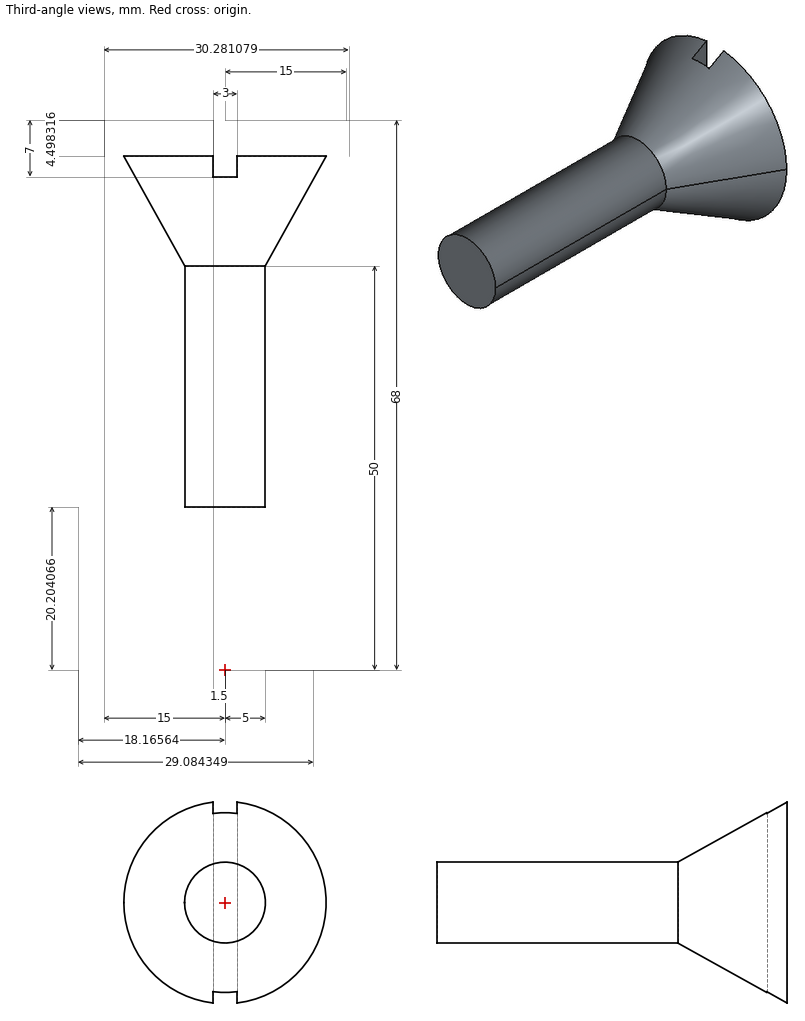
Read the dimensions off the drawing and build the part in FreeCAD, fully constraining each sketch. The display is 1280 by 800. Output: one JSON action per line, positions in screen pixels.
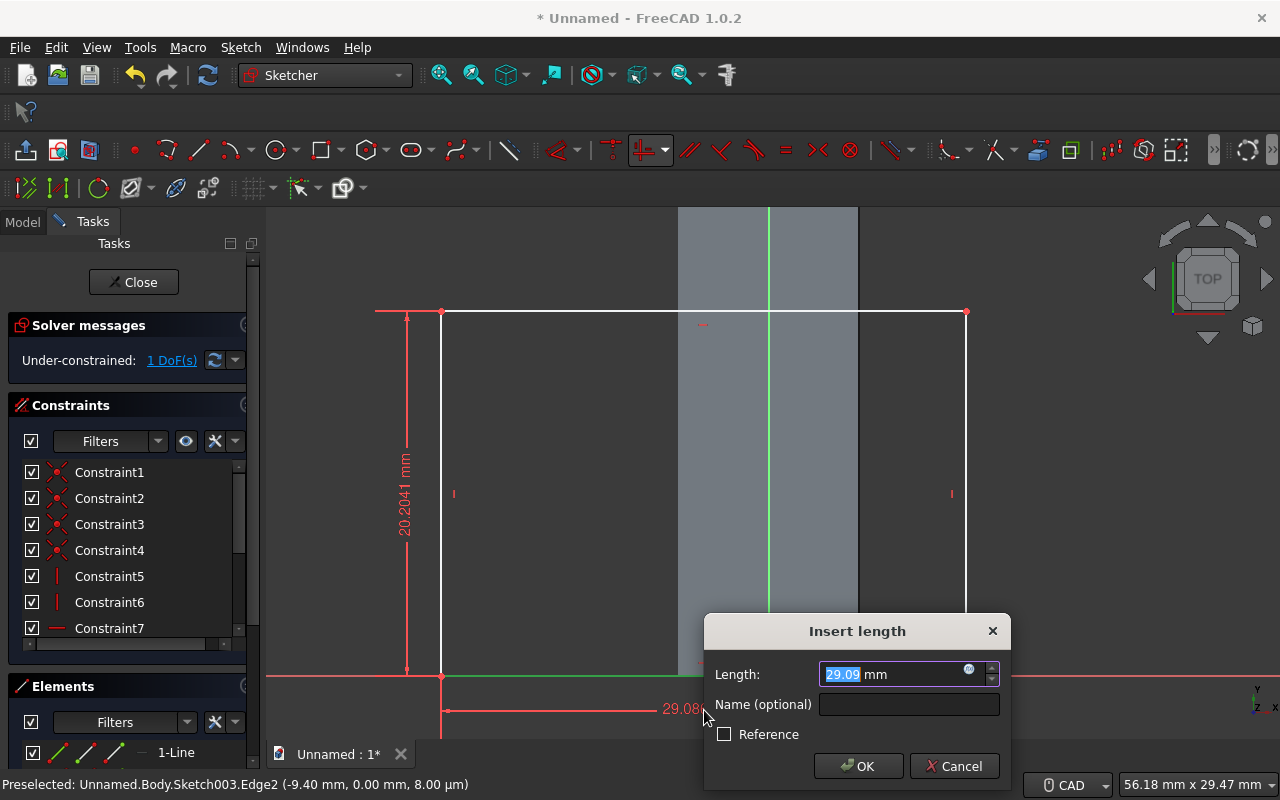
{"action": "type", "text": "29.084349"}
{"action": "key", "text": "Return"}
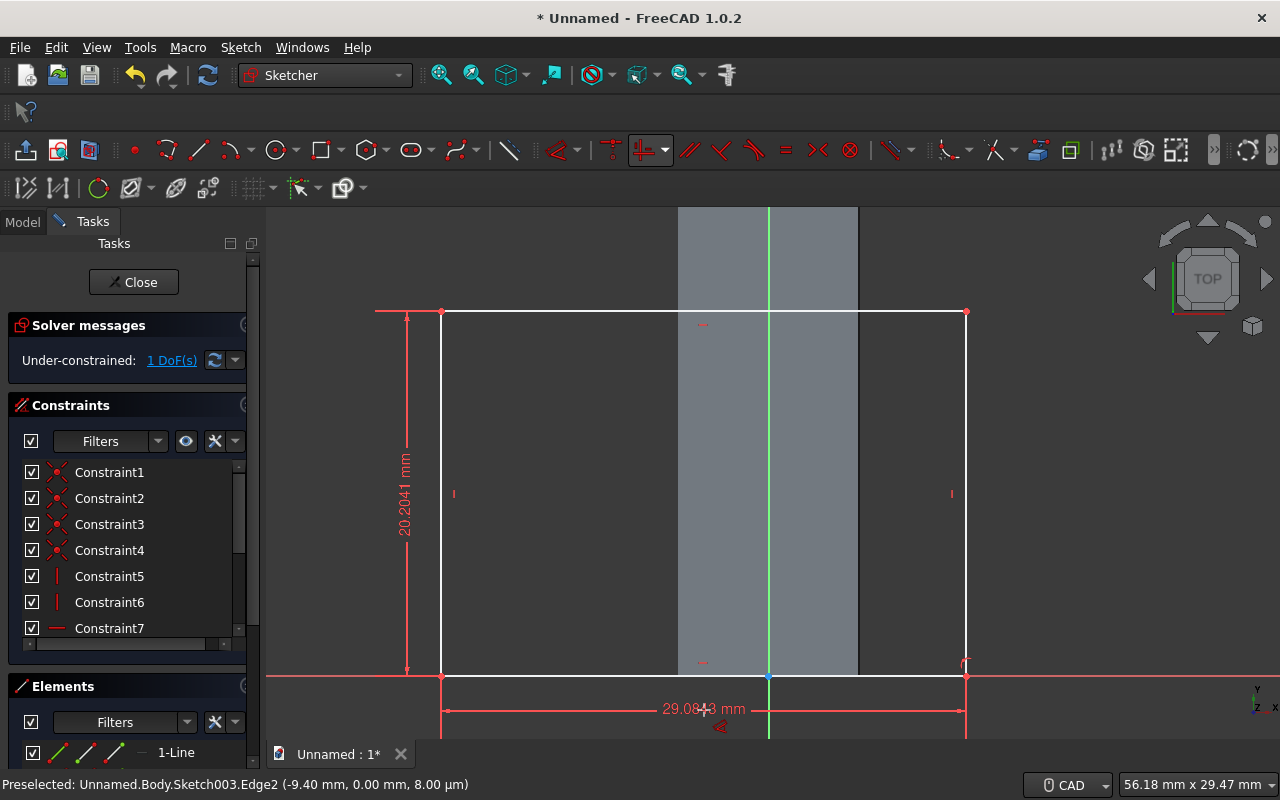
{"action": "left_click", "coordinate": [441, 311]}
{"action": "left_click", "coordinate": [605, 277]}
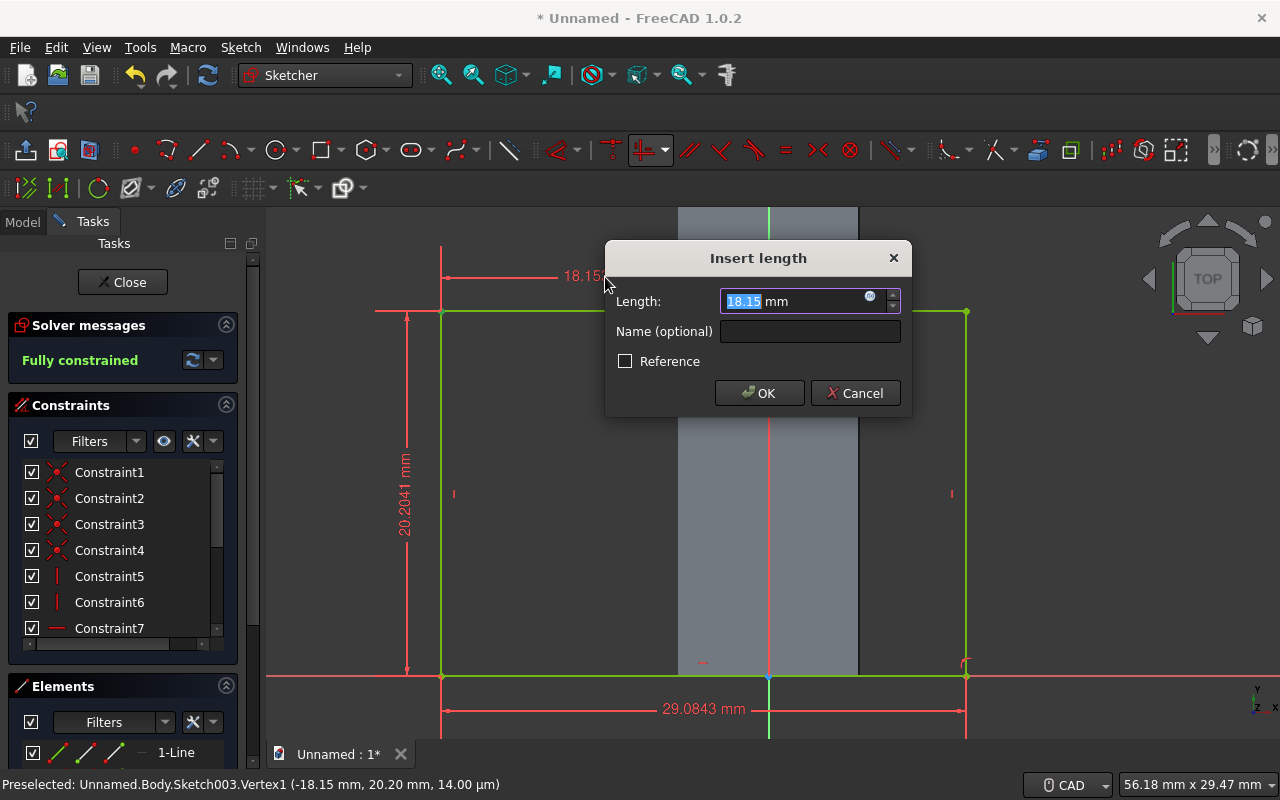
{"action": "type", "text": "18.16564"}
{"action": "key", "text": "Return"}
{"action": "key", "text": "Escape"}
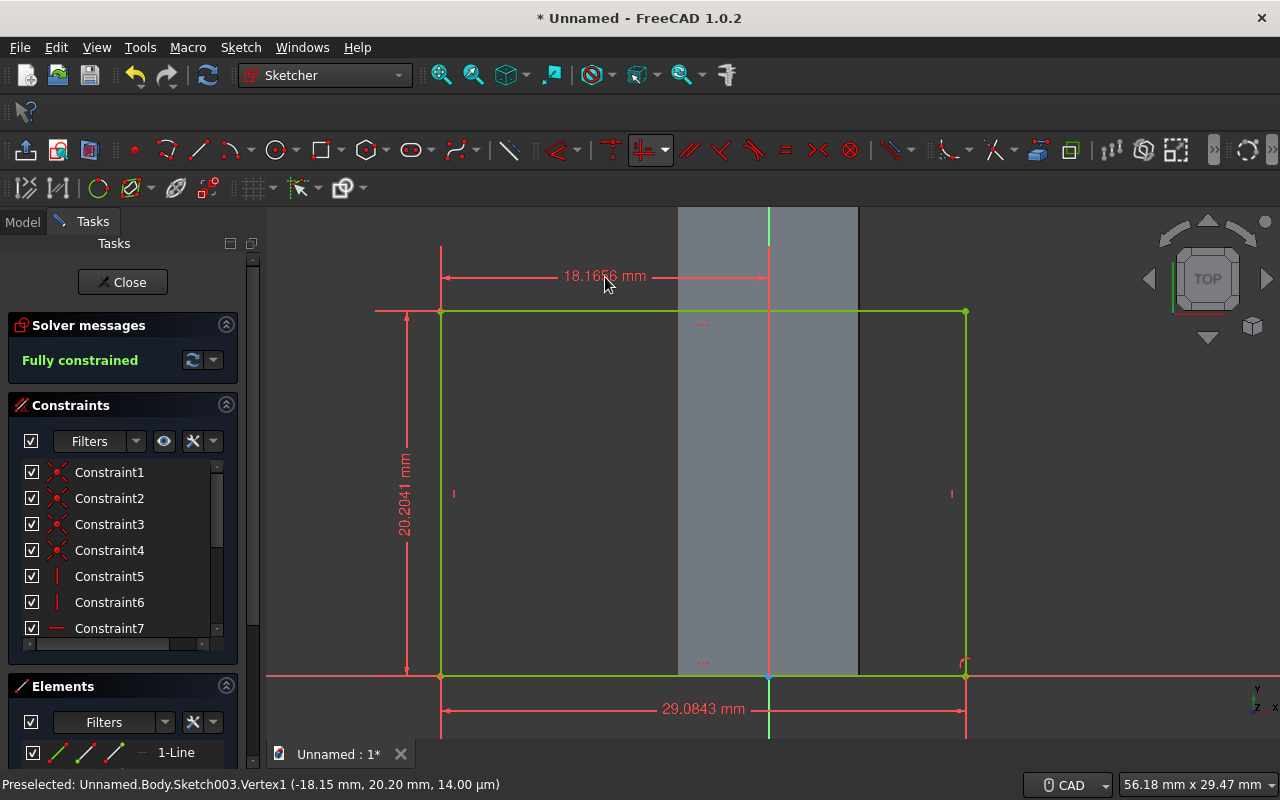
{"action": "left_click", "coordinate": [123, 282]}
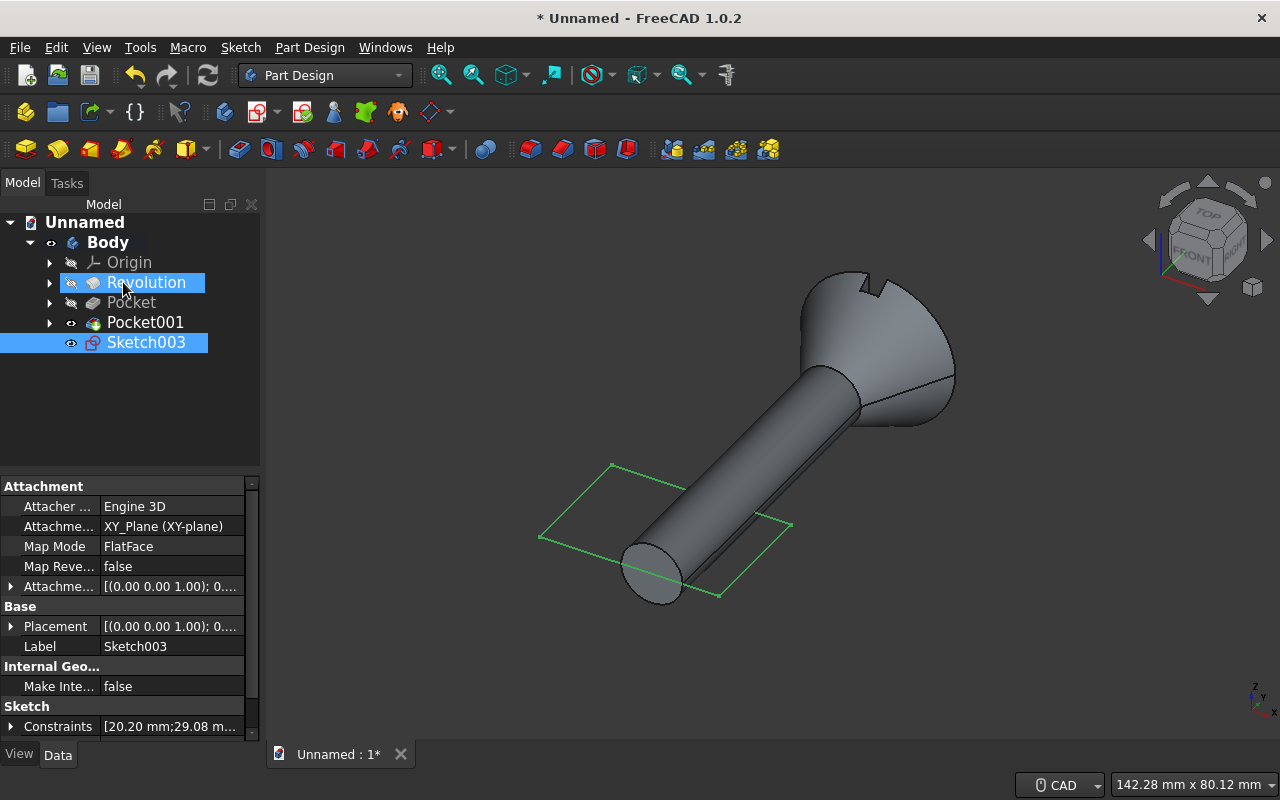
{"action": "left_click", "coordinate": [240, 150]}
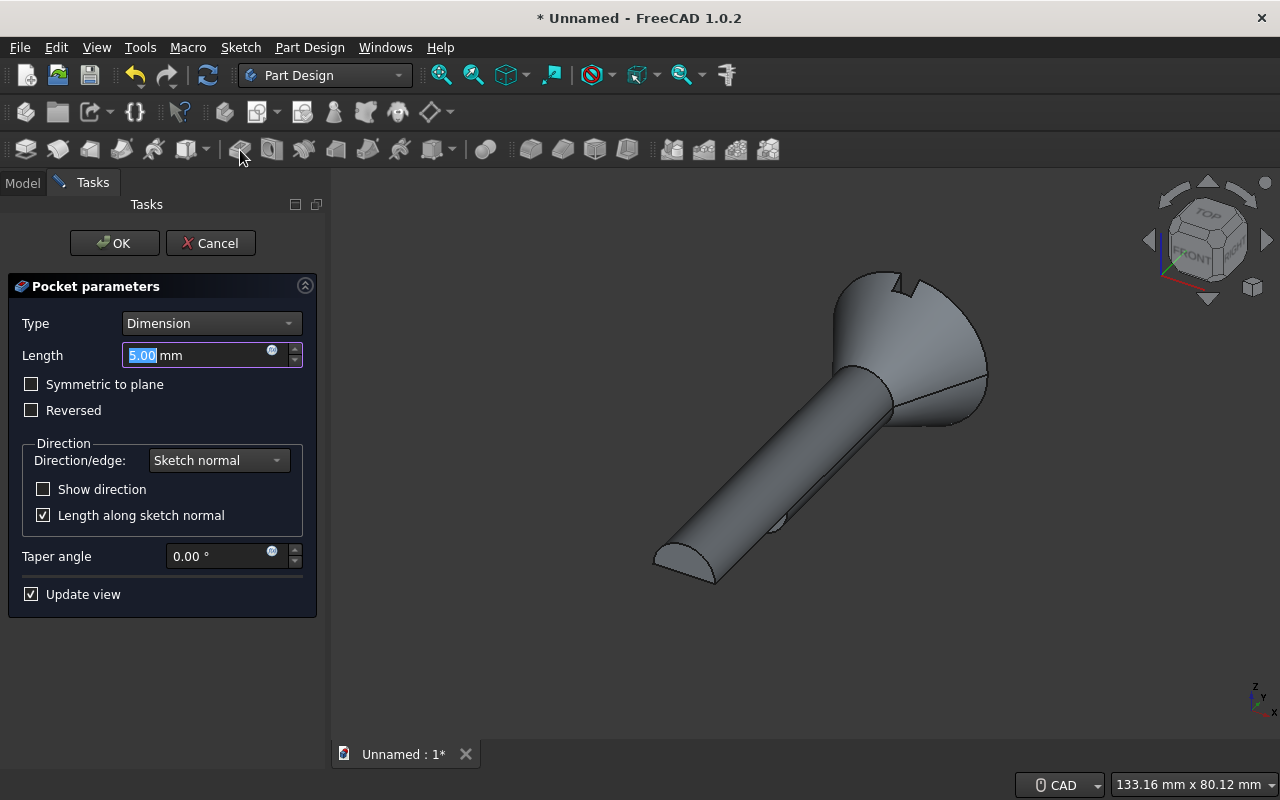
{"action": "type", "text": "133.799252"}
{"action": "key", "text": "Tab"}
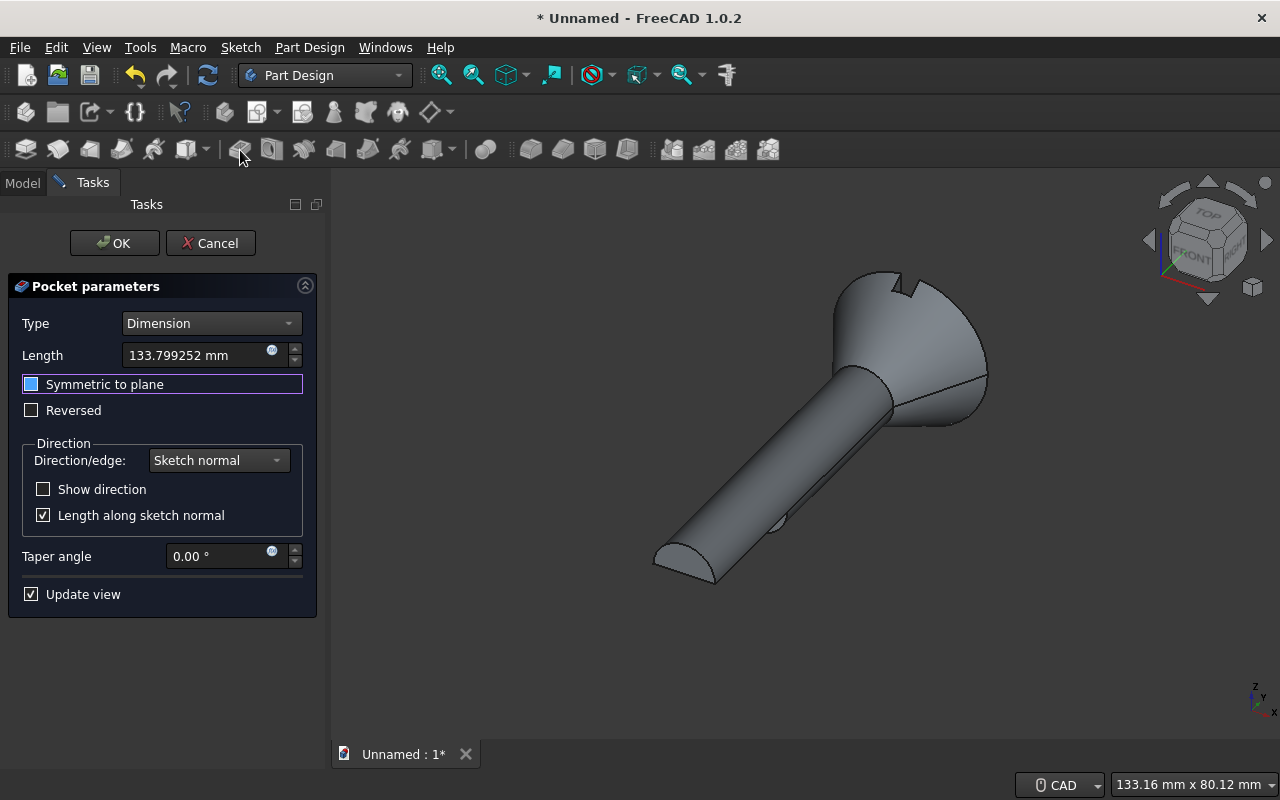
{"action": "left_click", "coordinate": [30, 384]}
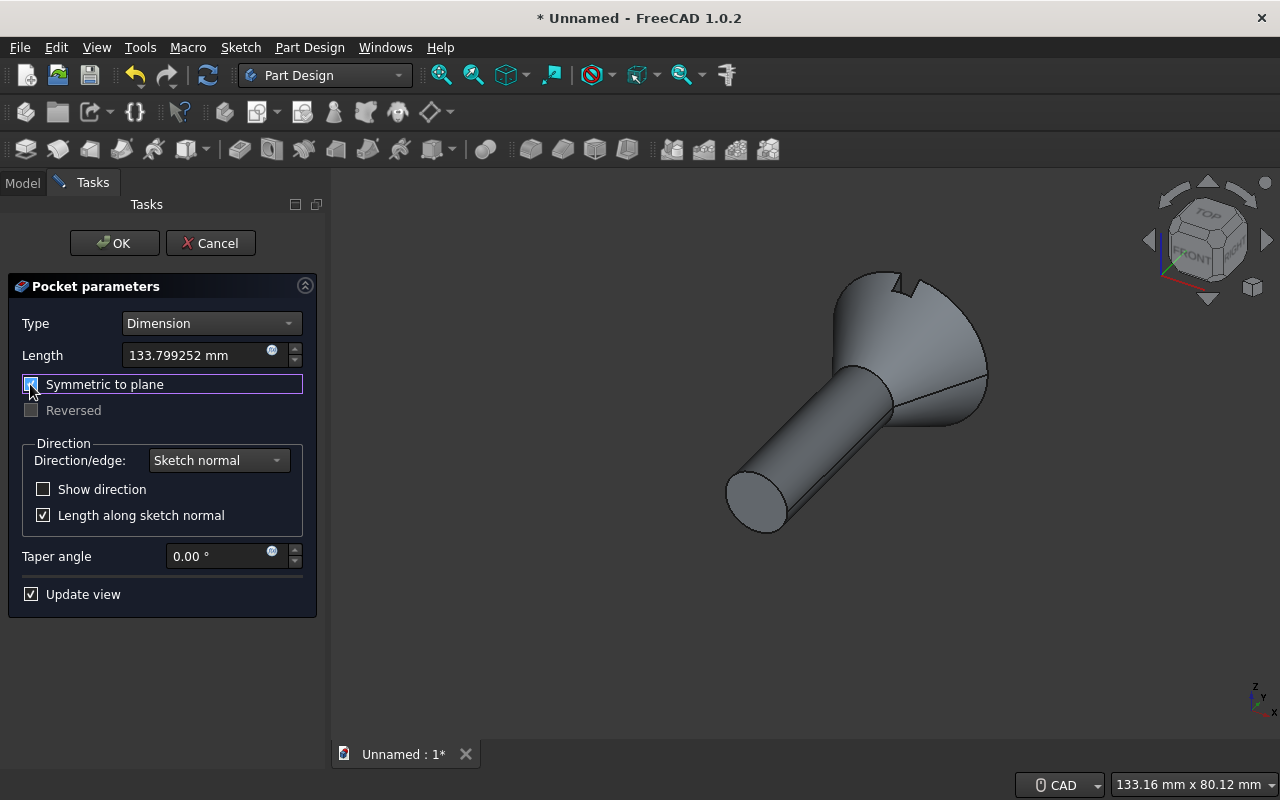
{"action": "left_click", "coordinate": [115, 243]}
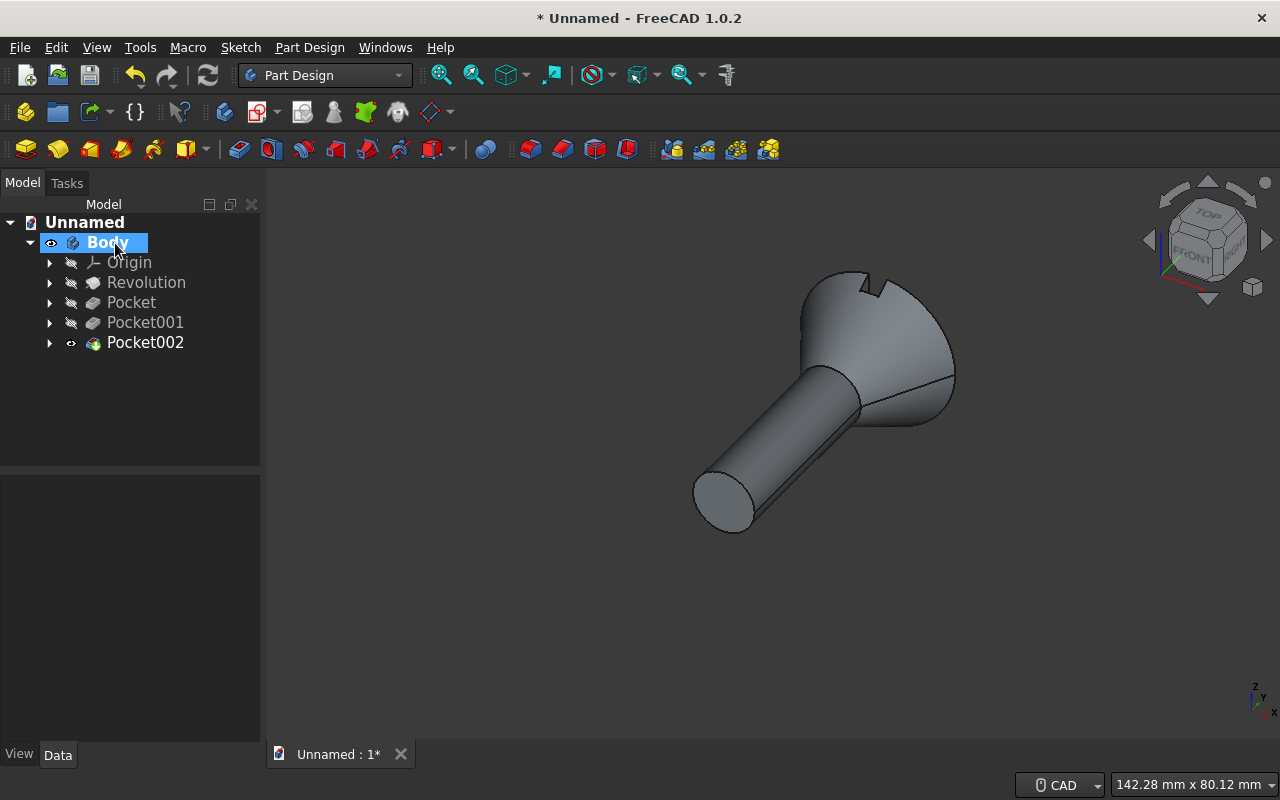
{"action": "key", "text": "0"}